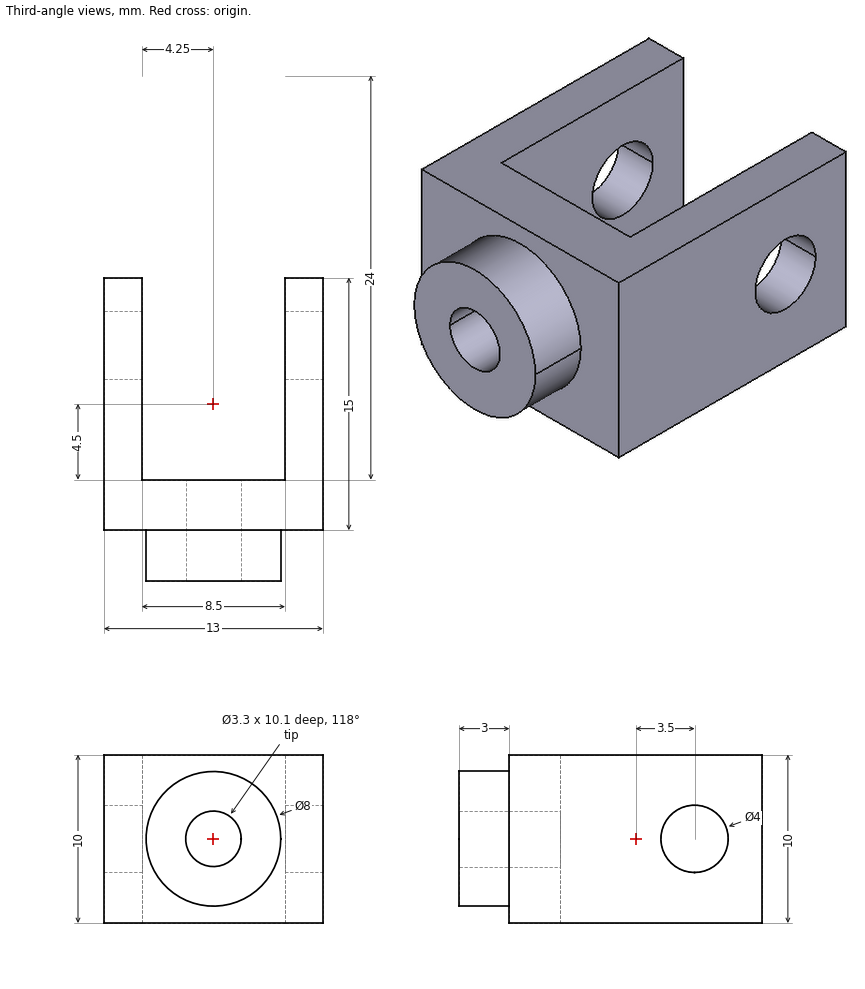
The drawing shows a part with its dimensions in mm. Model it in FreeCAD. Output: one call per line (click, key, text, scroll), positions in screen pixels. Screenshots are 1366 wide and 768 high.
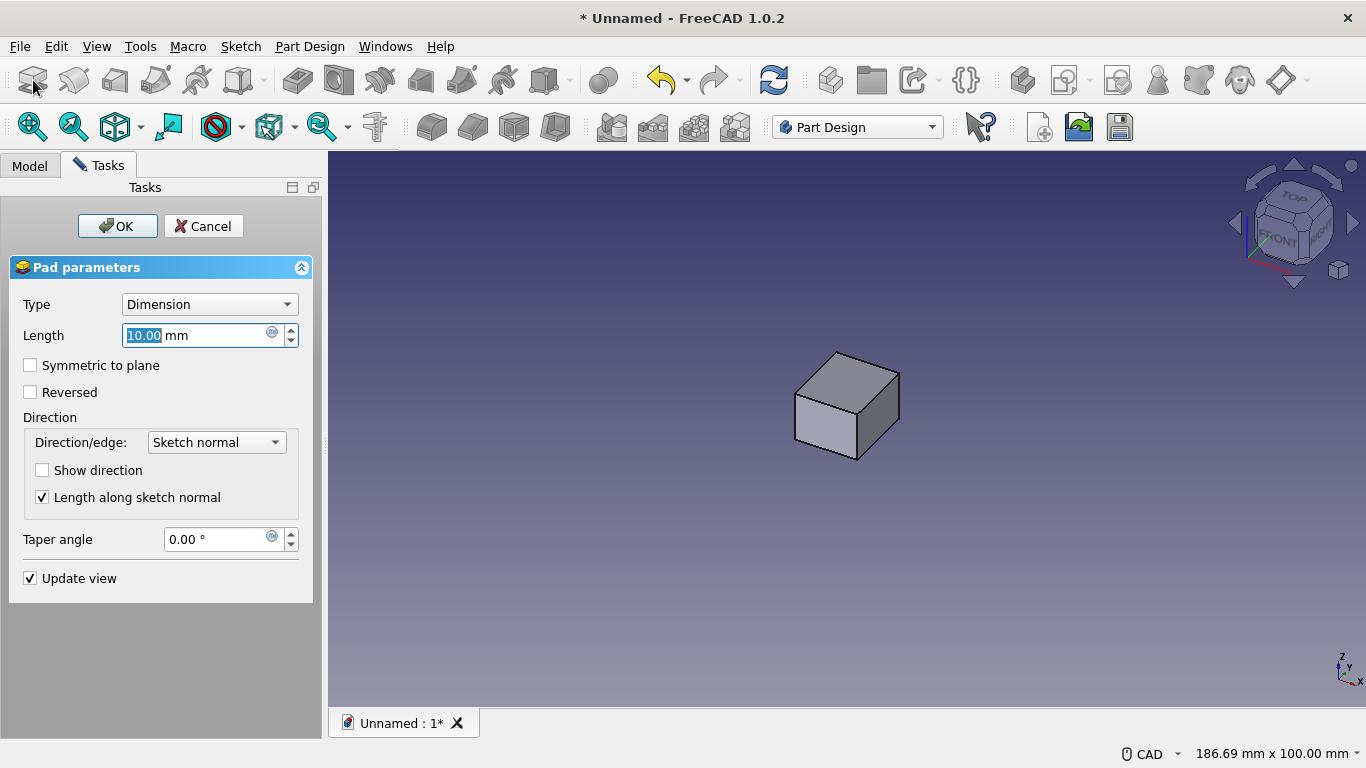
text(10)
key(Tab)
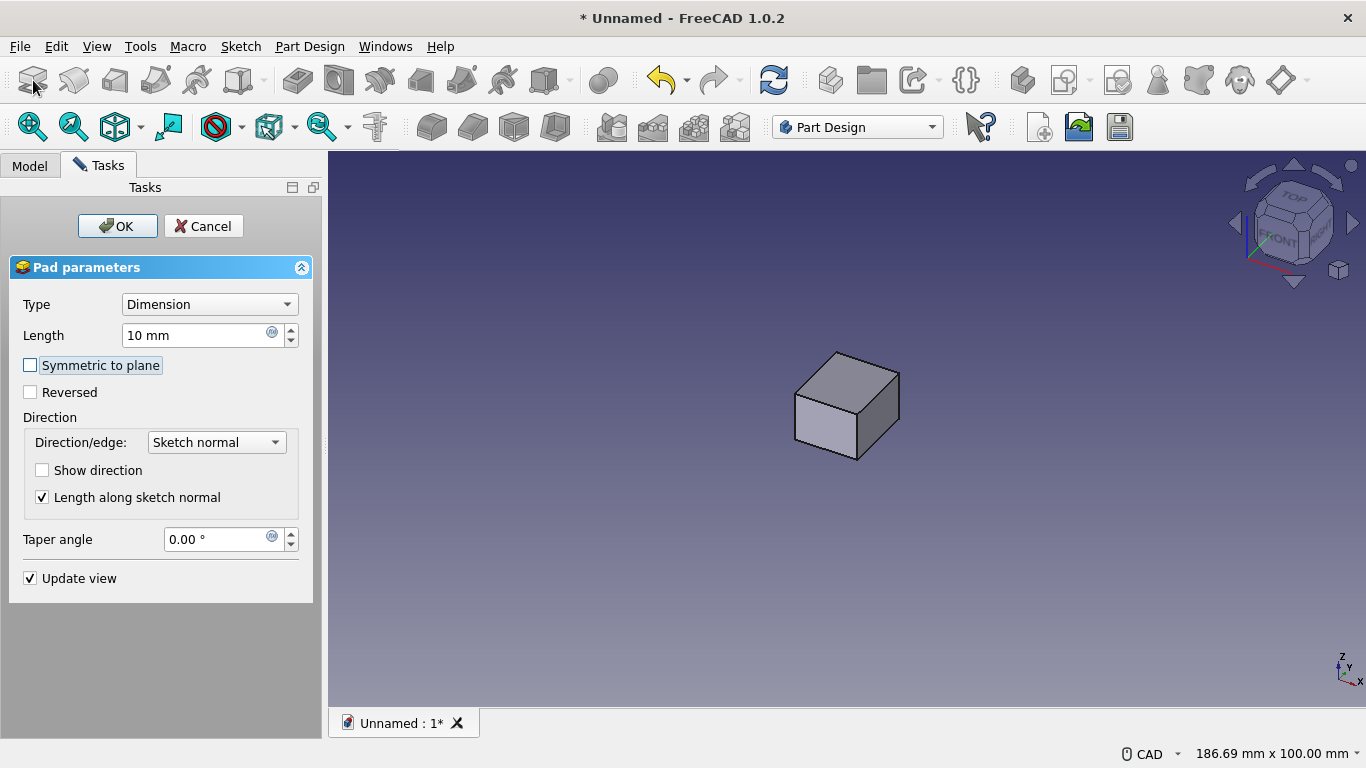
click(31, 365)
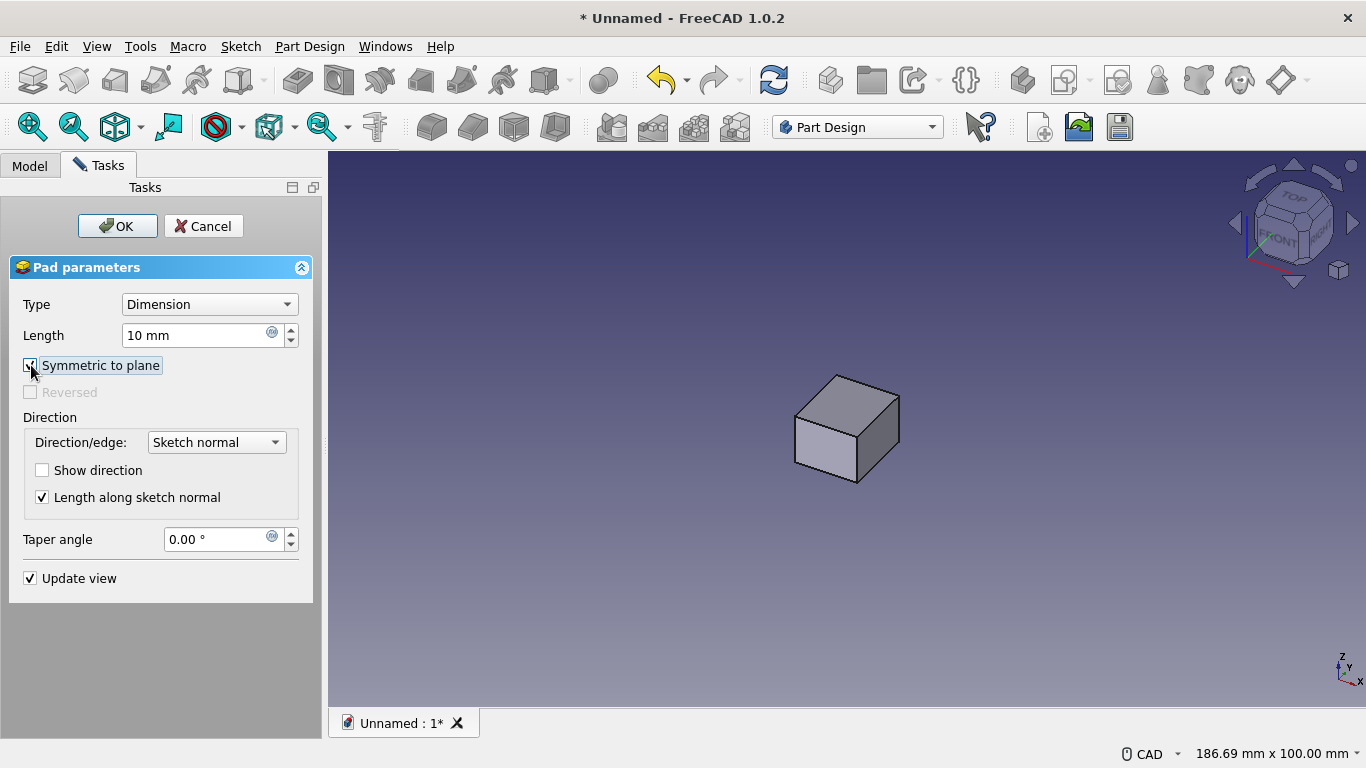
click(118, 226)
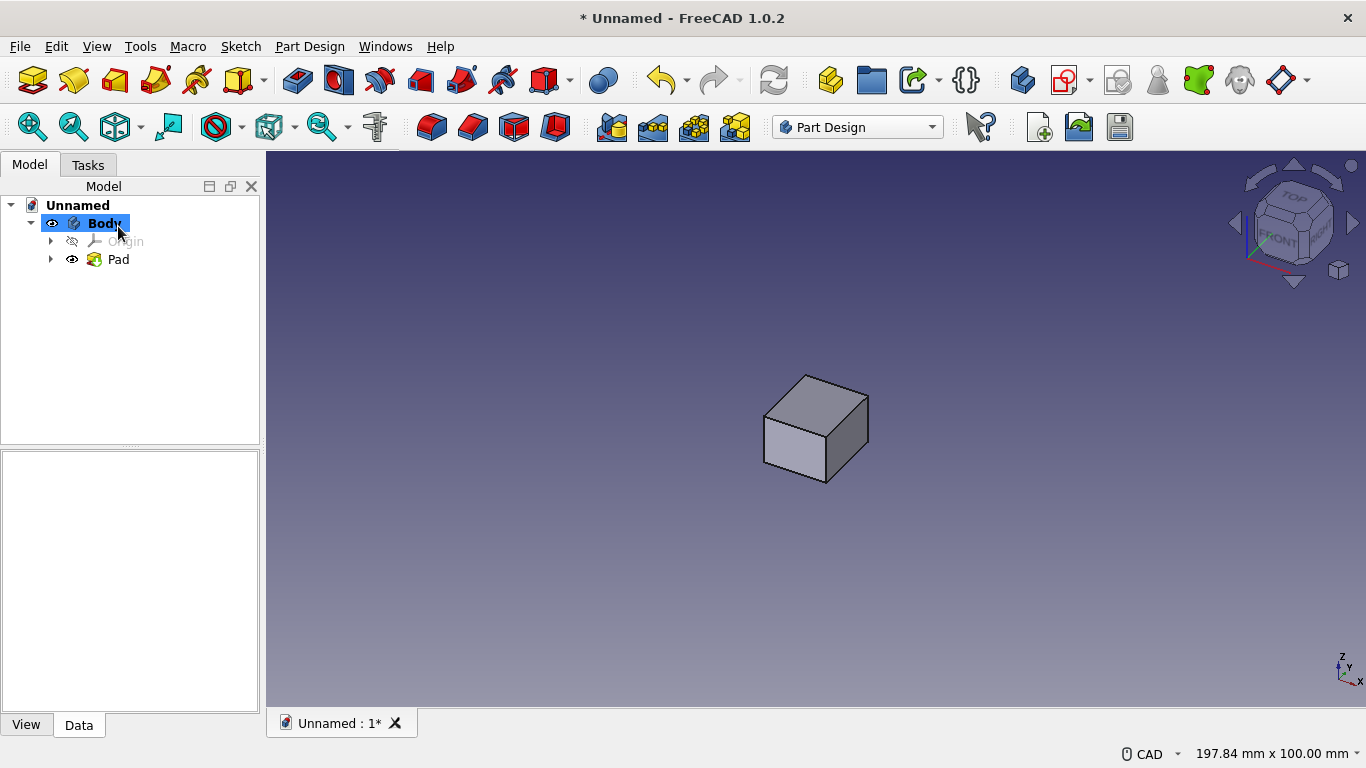
click(33, 128)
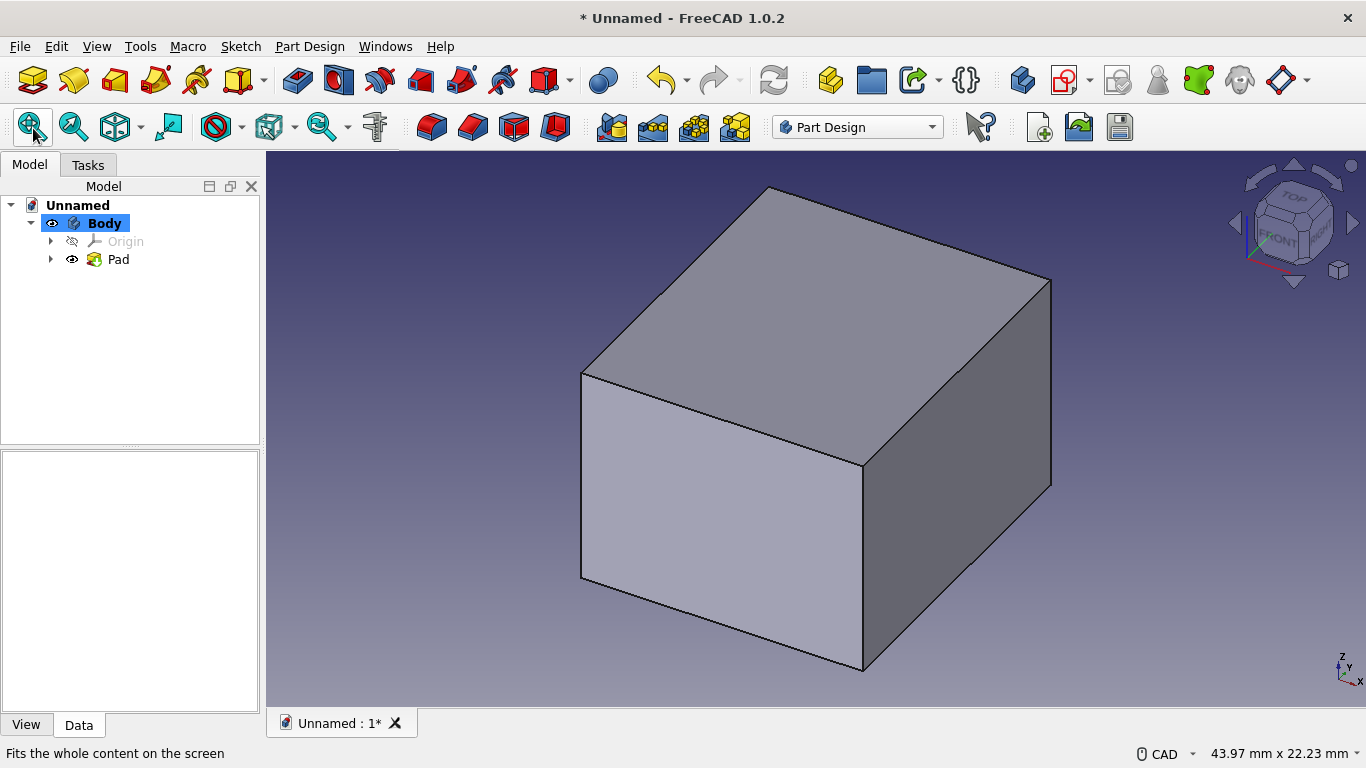
click(816, 326)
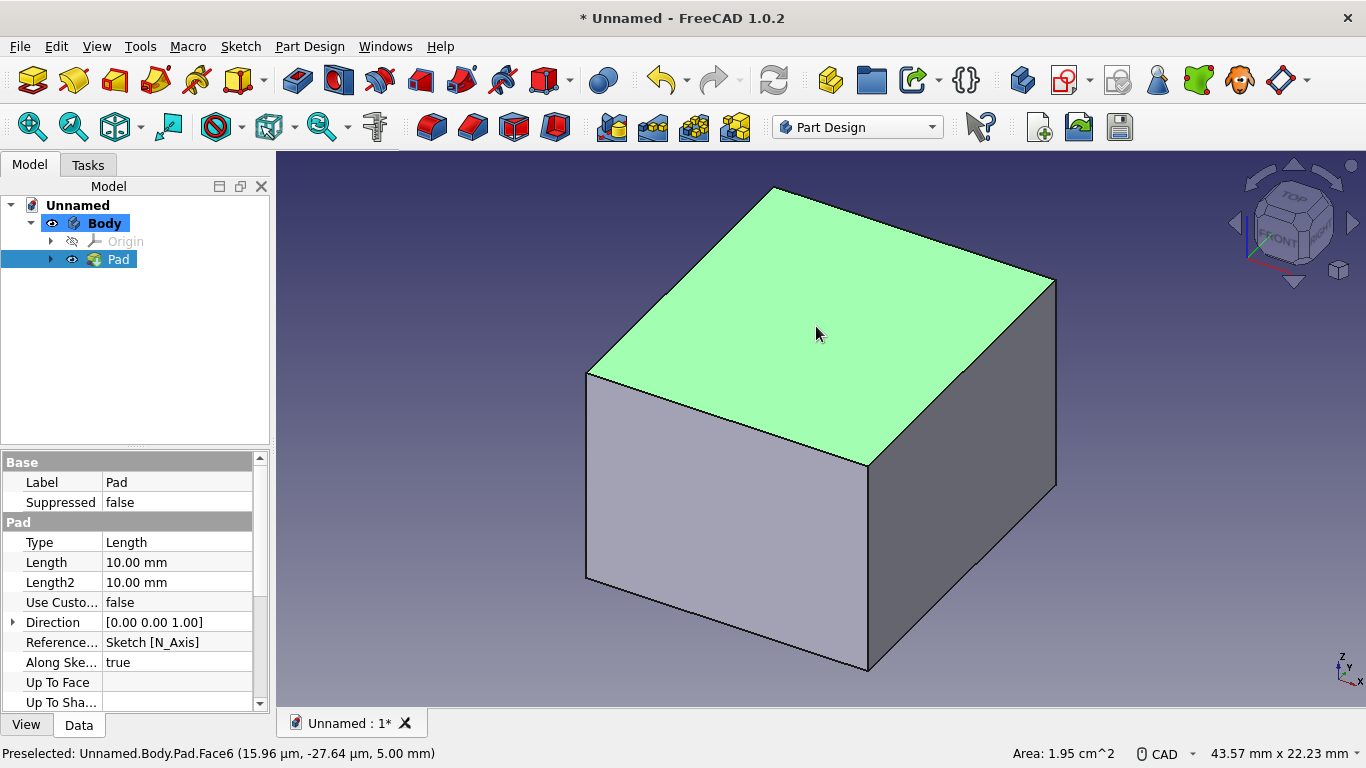
click(1064, 80)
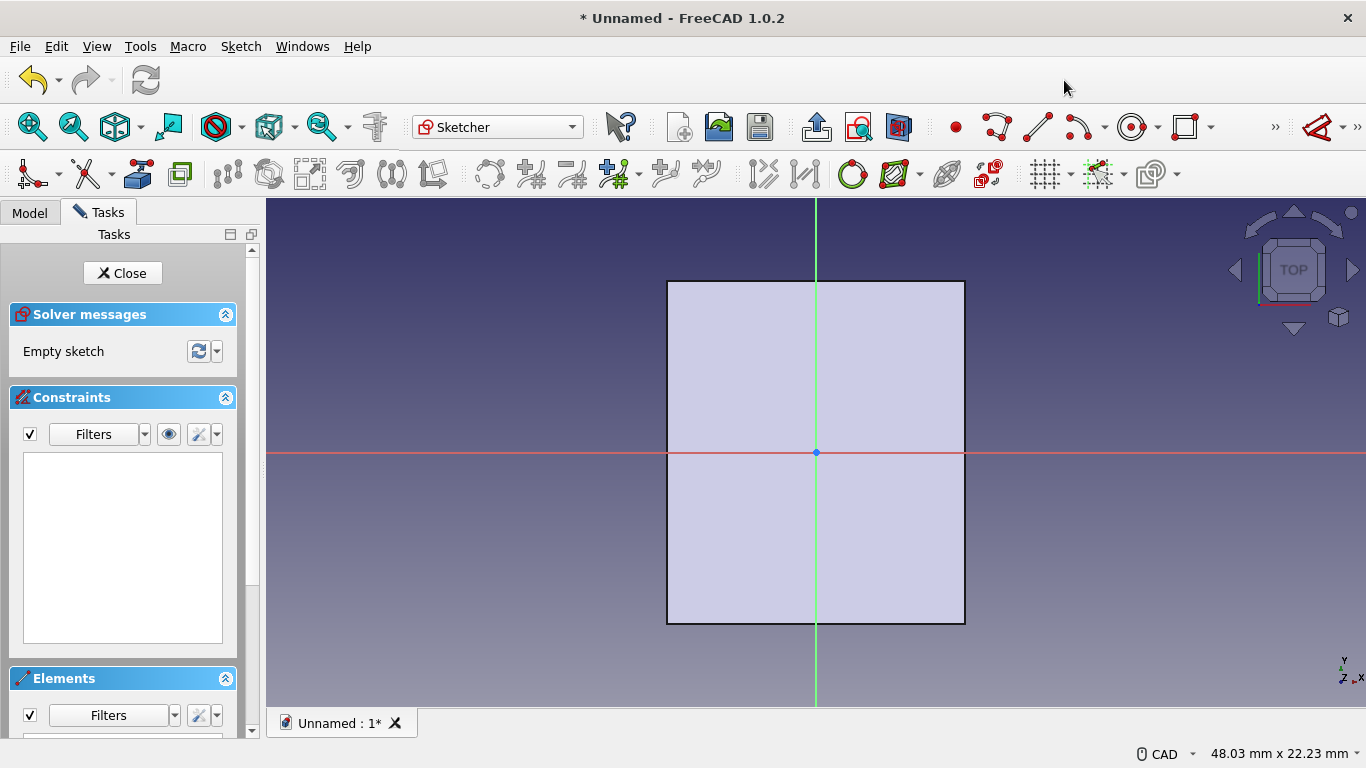
scroll(664, 661, down, 3)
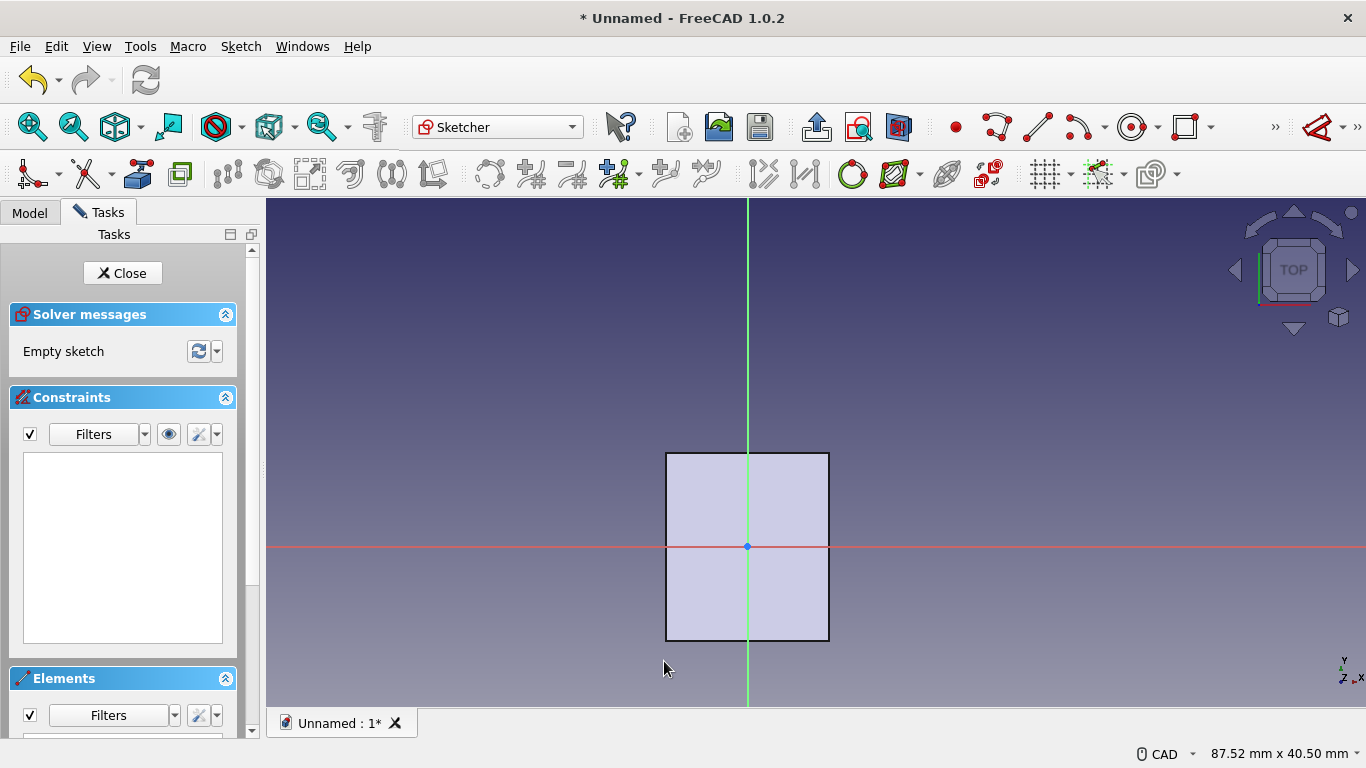
key(g)
key(r)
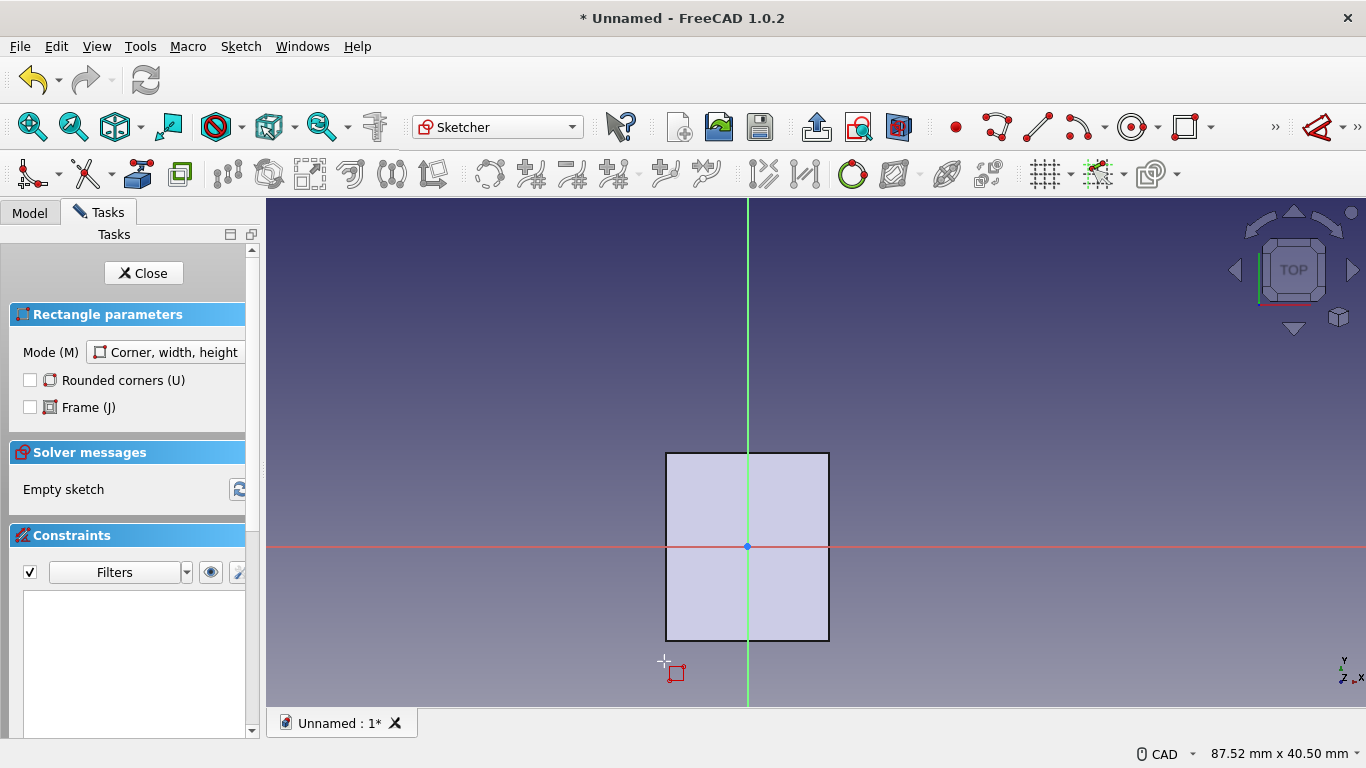
click(694, 302)
move(801, 604)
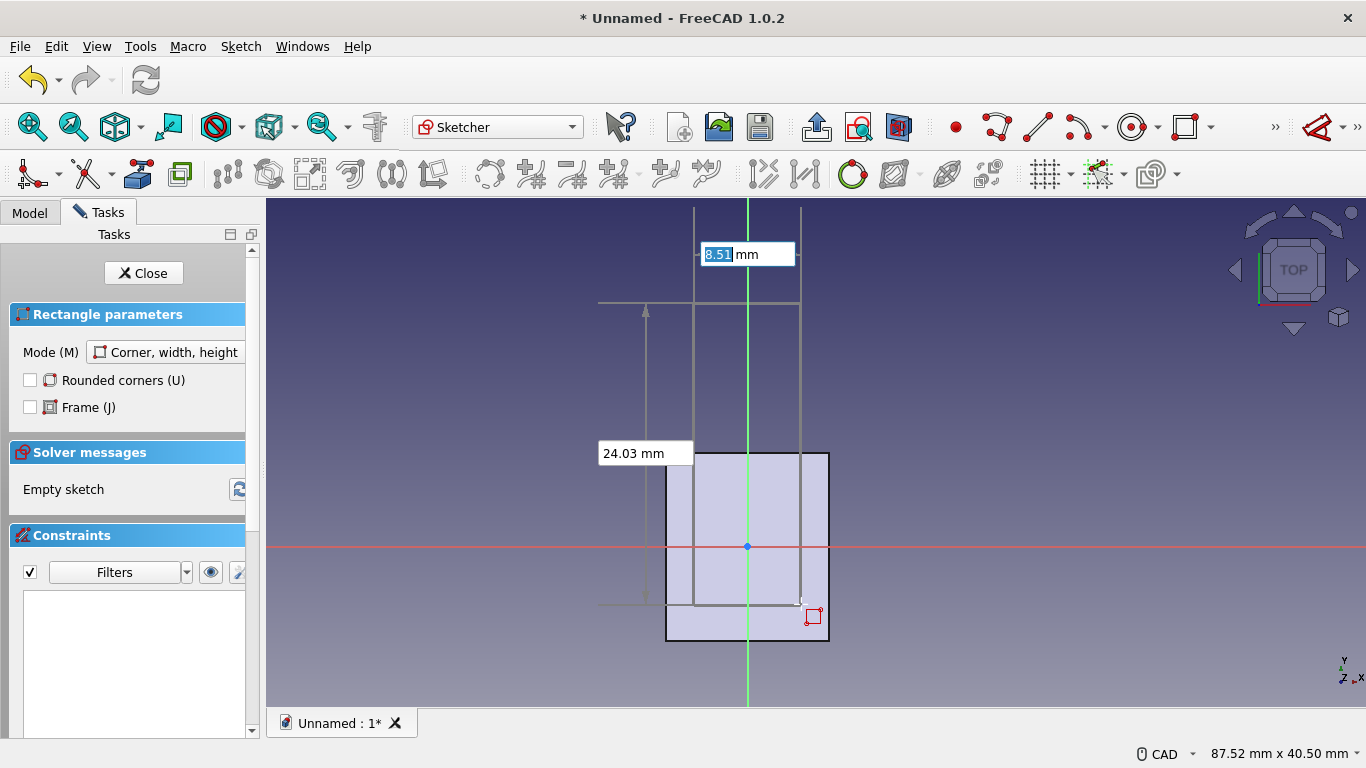
text(8.5)
key(Tab)
text(24)
key(Return)
key(Escape)